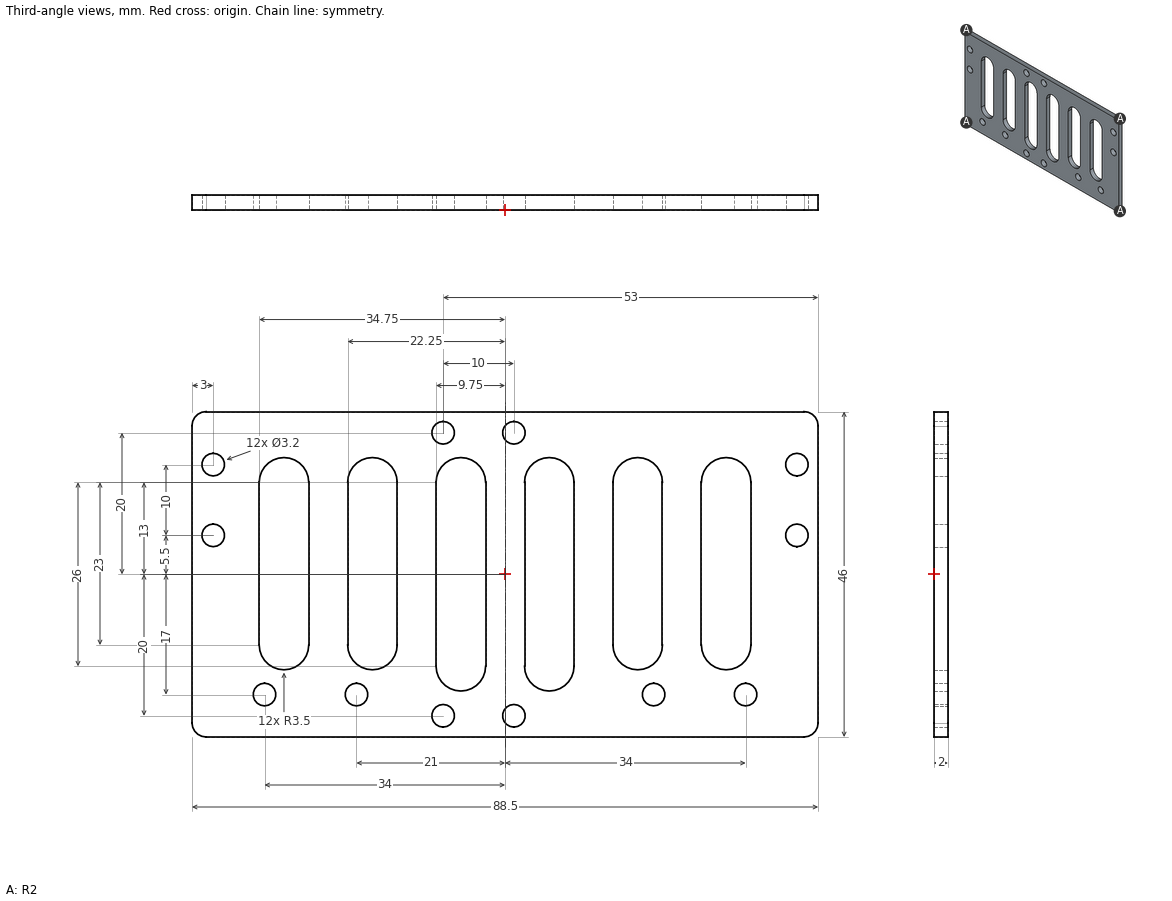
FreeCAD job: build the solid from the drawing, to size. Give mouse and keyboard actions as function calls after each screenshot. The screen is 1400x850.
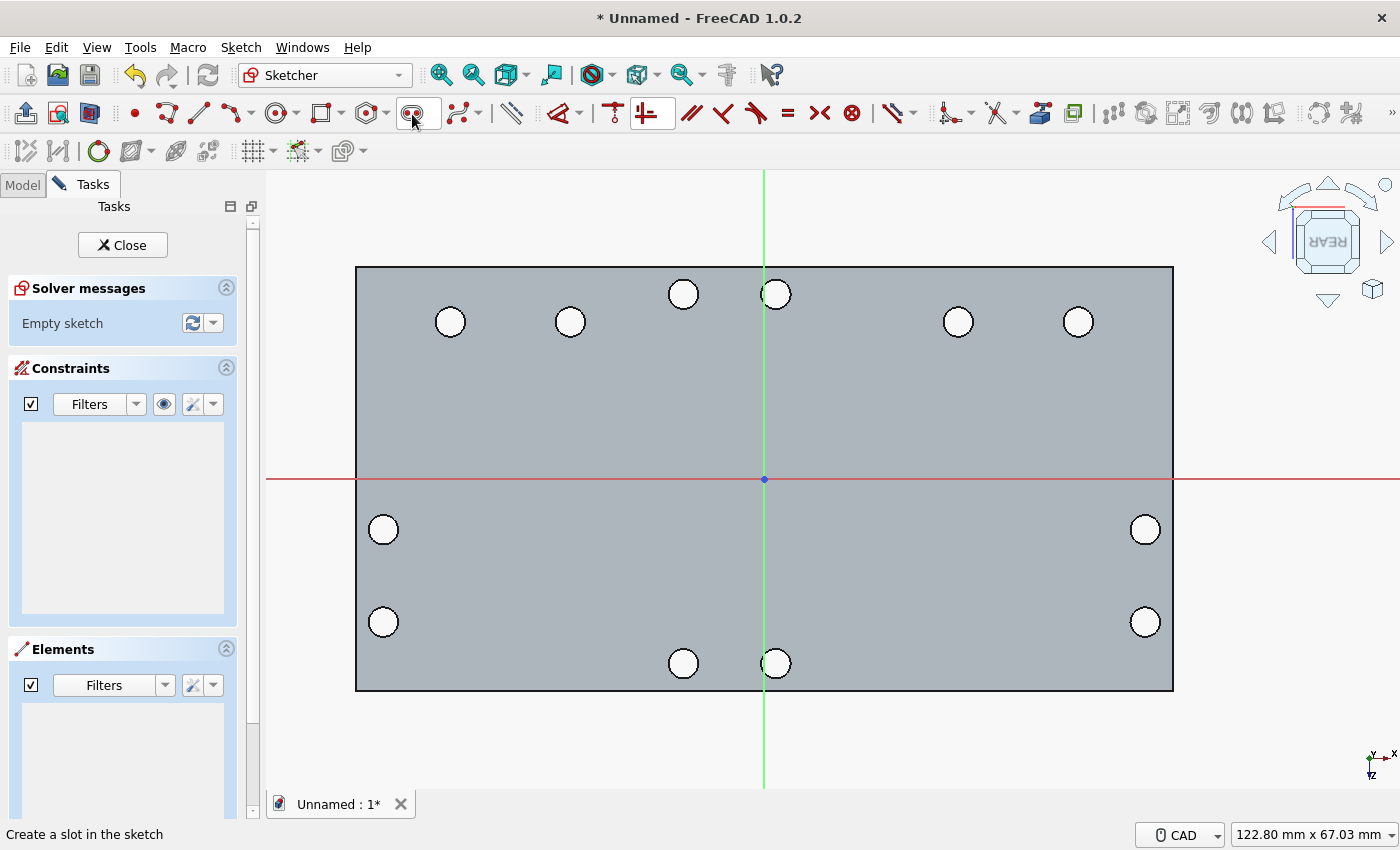
click(476, 599)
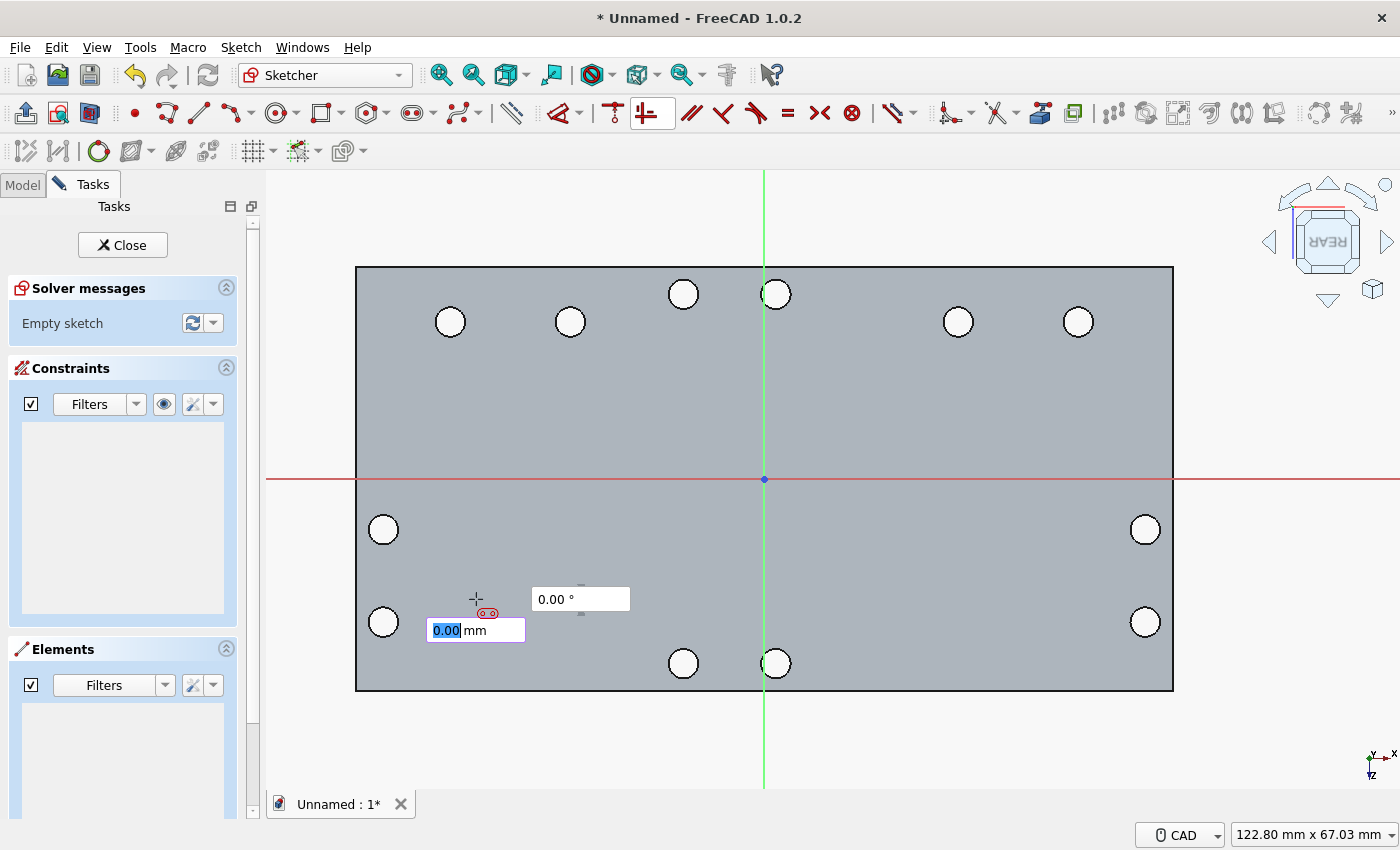
click(476, 387)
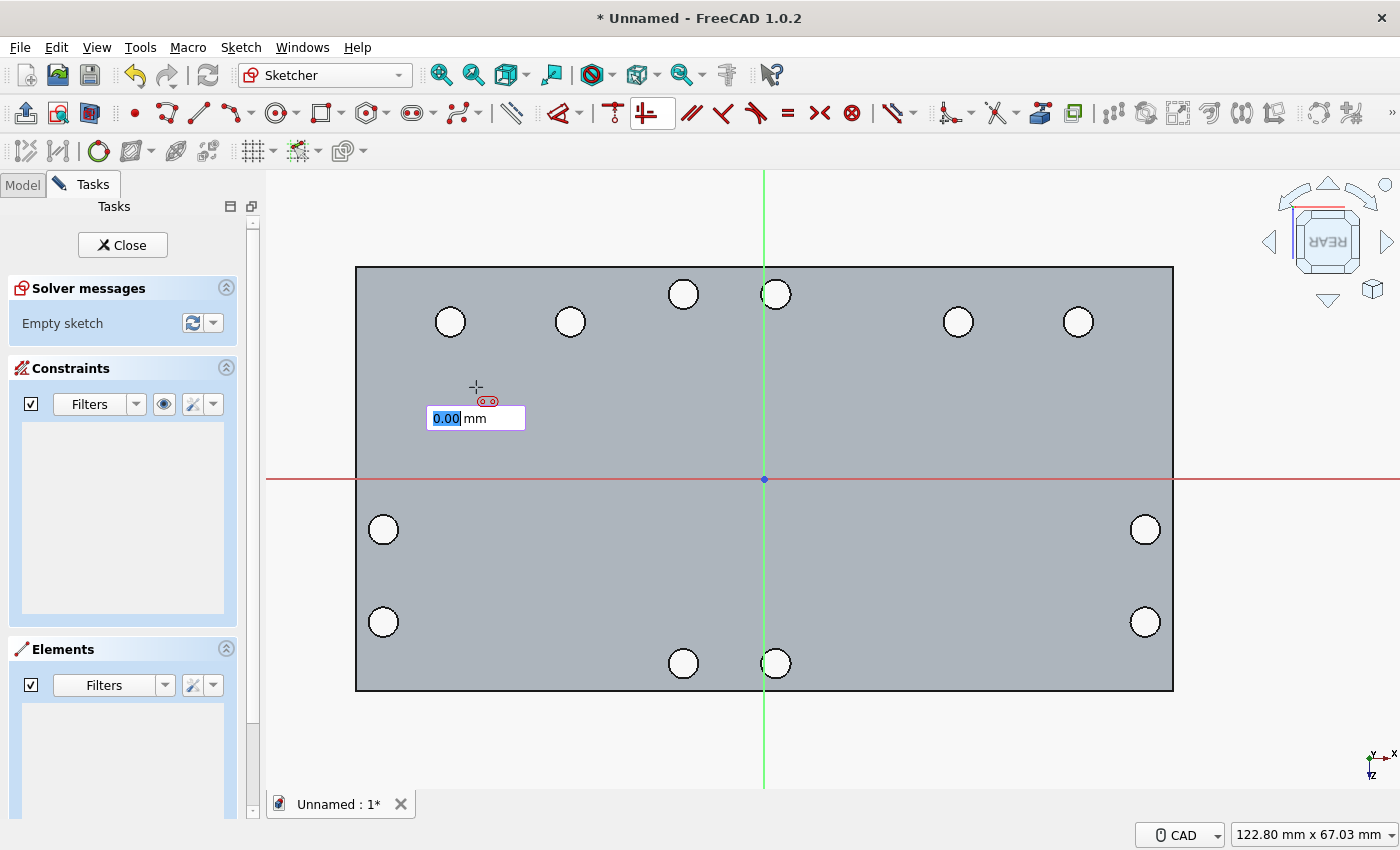
click(508, 525)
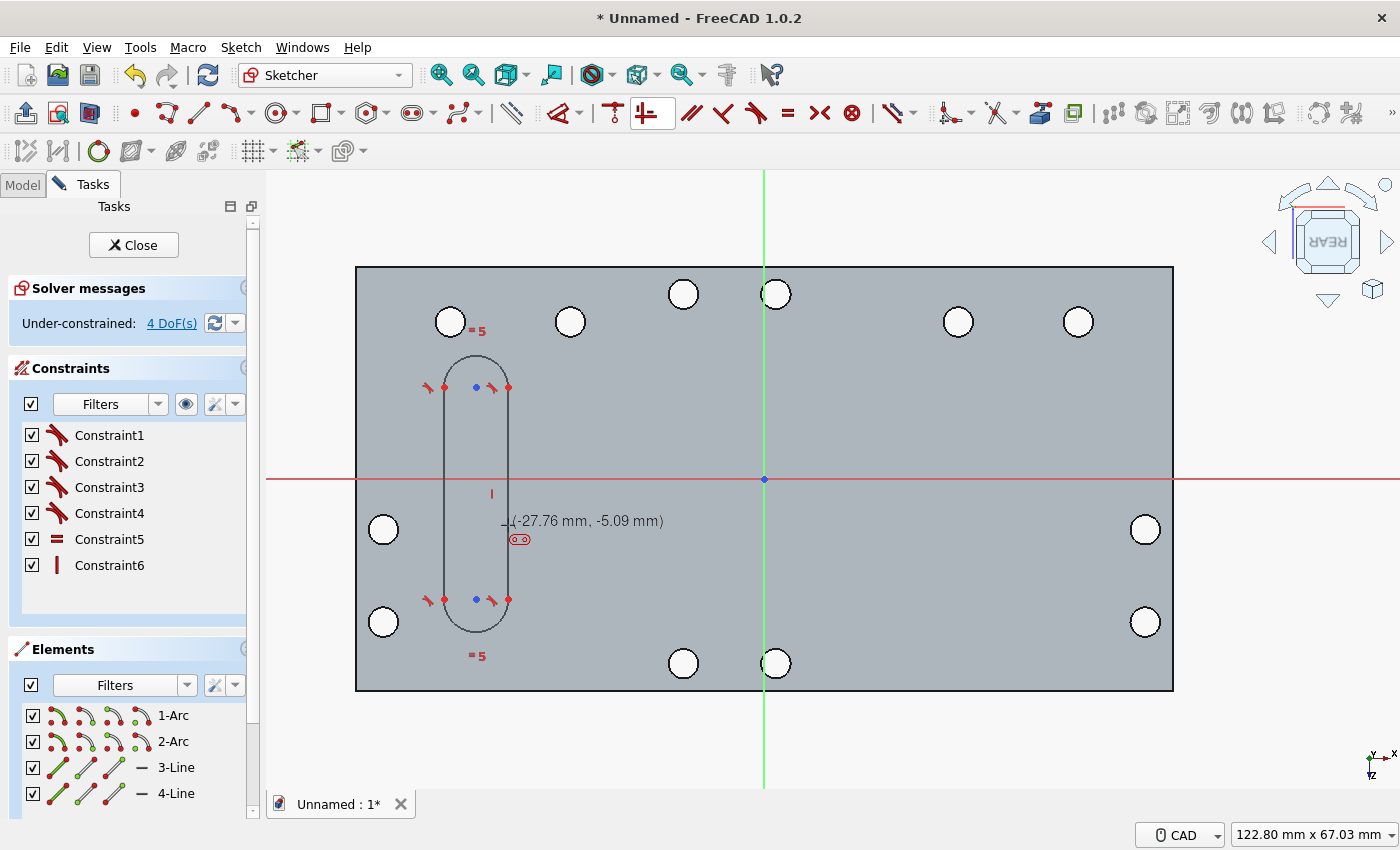
click(591, 599)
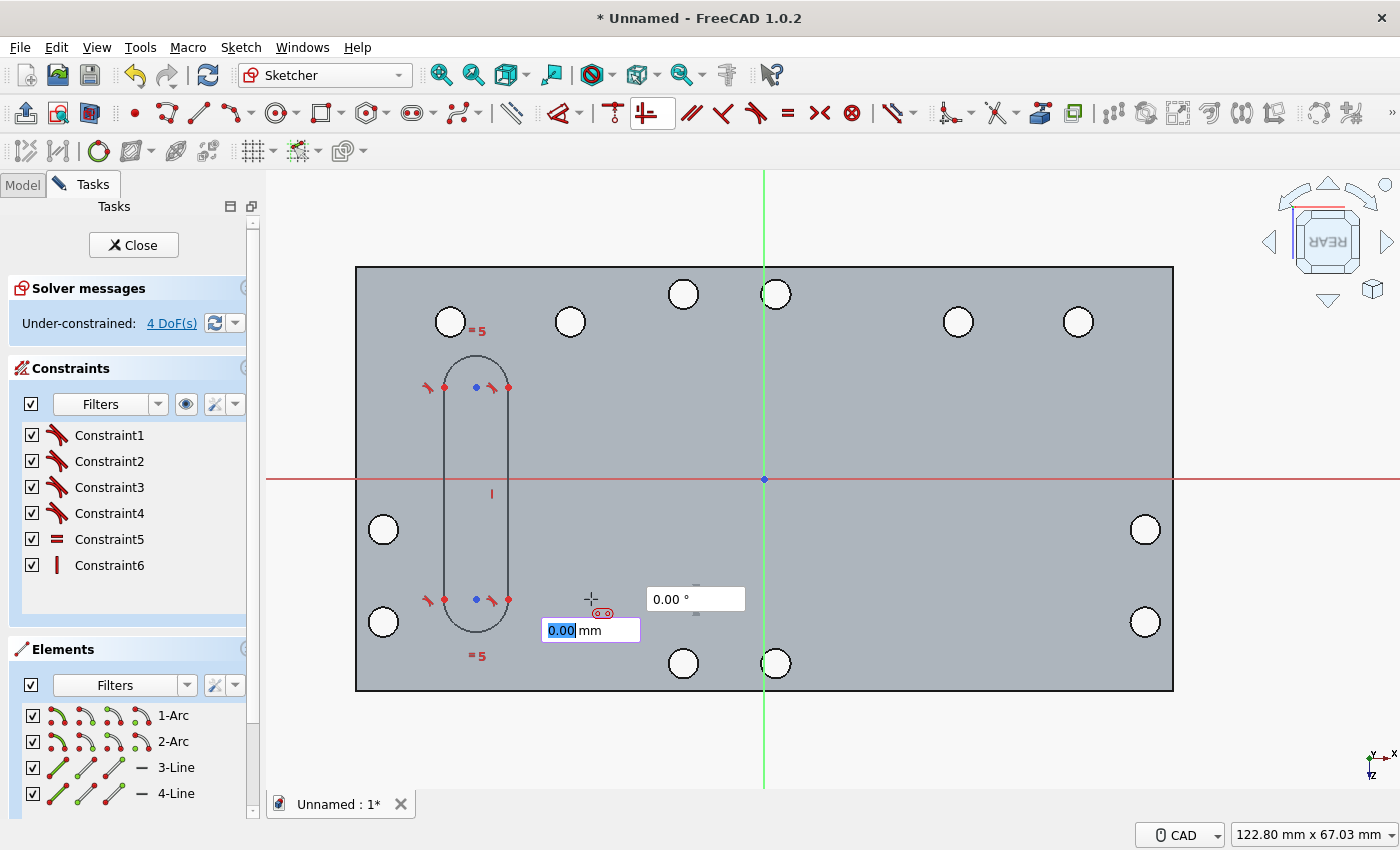
click(591, 387)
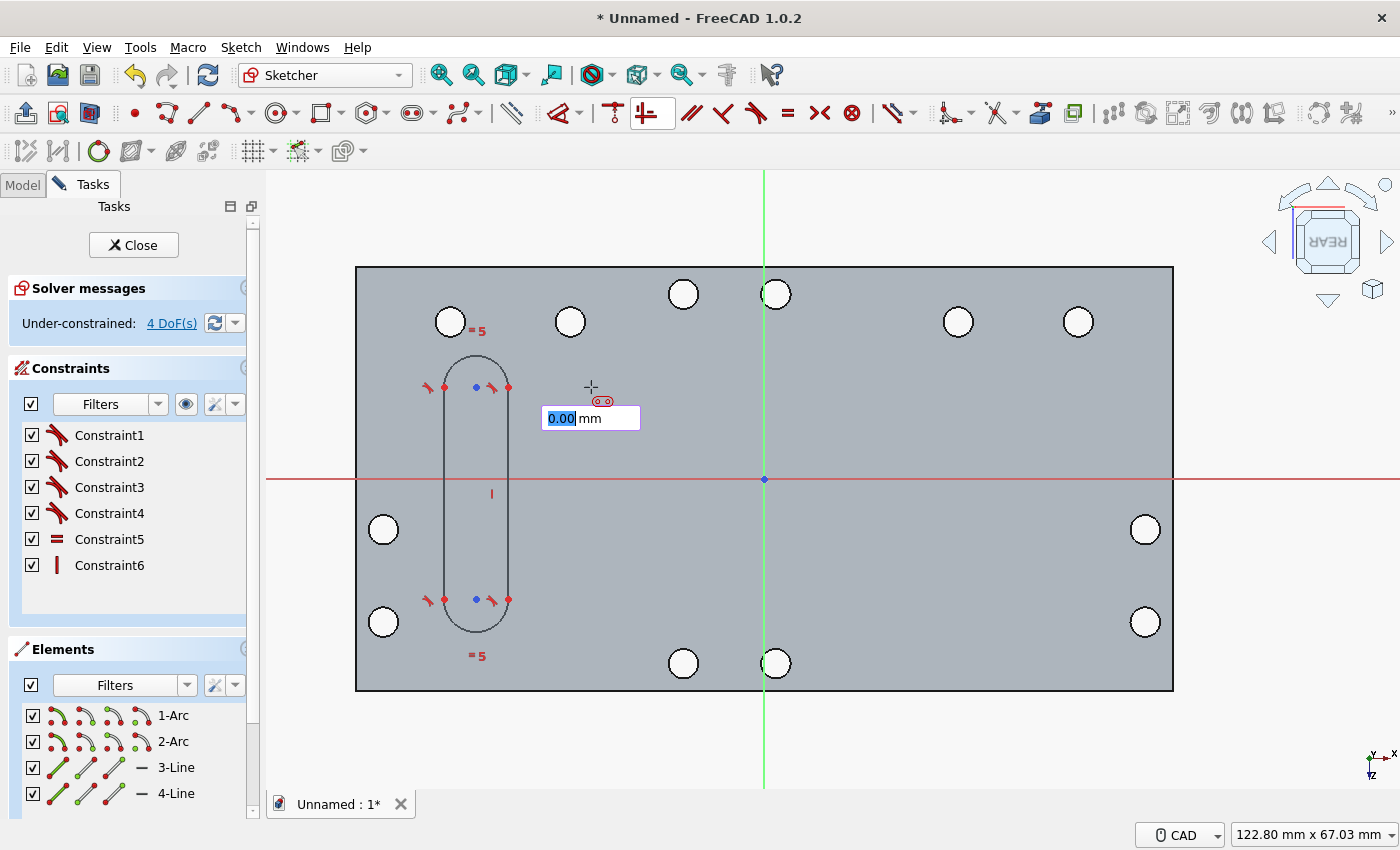
click(624, 525)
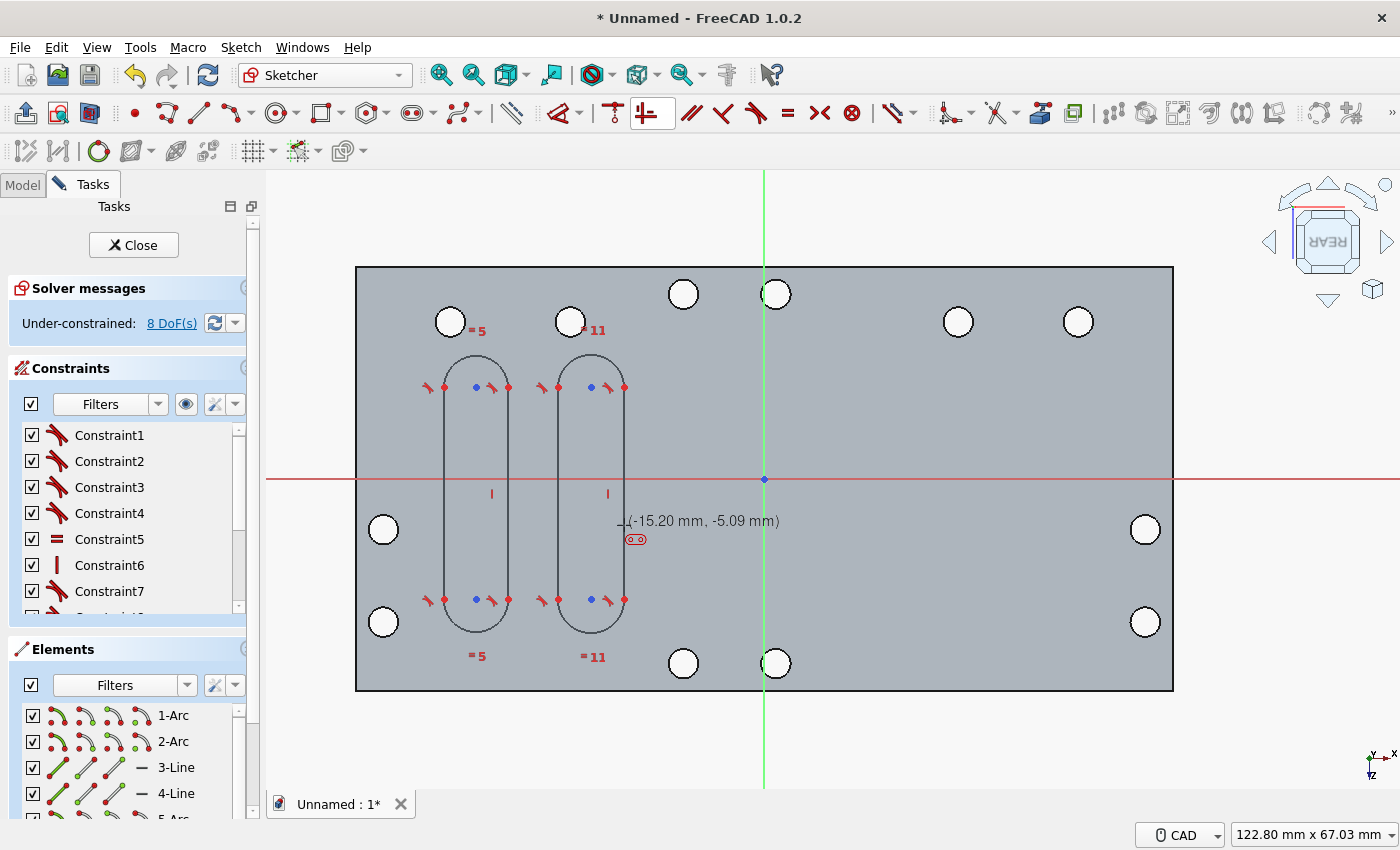
click(707, 599)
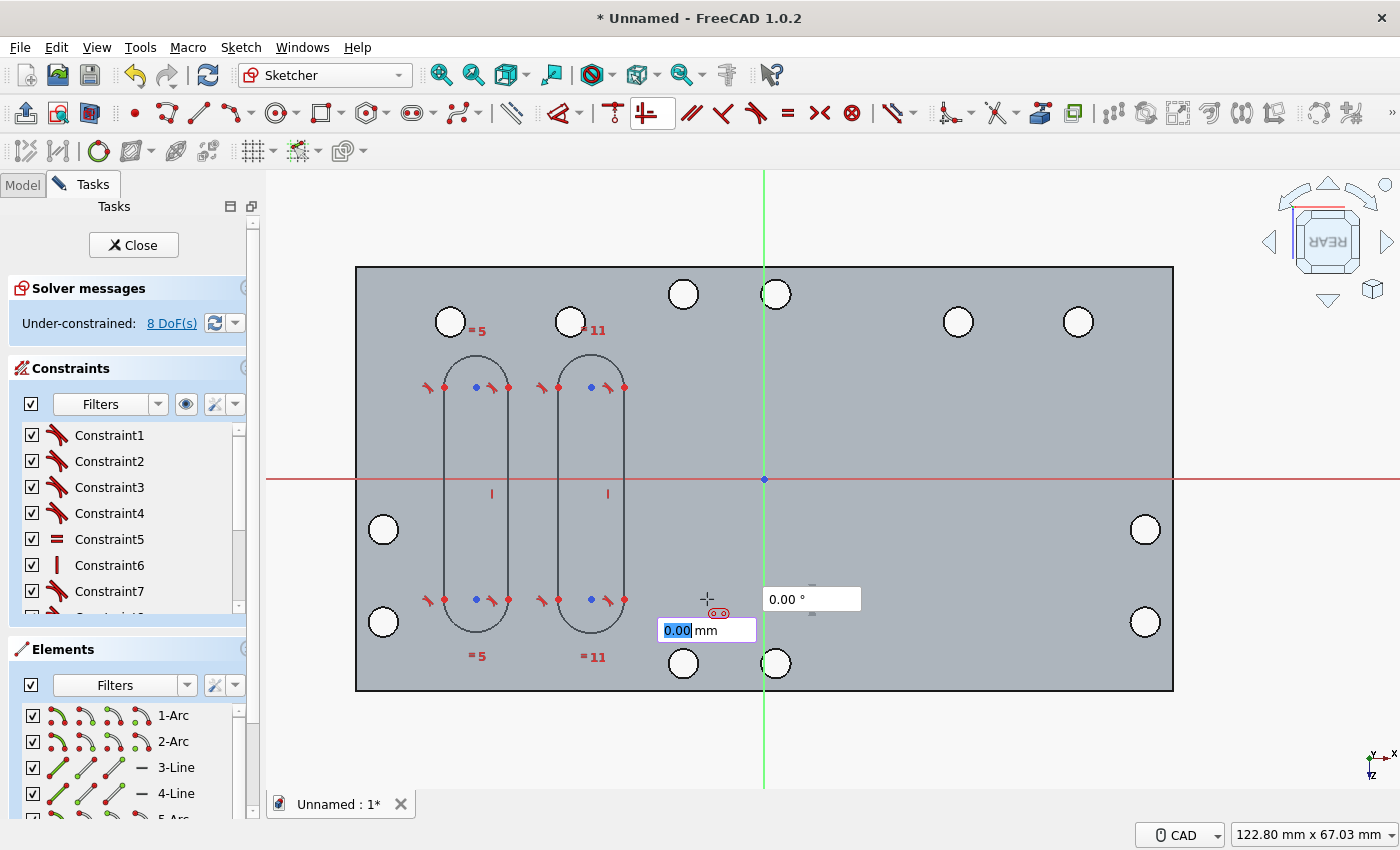
click(707, 359)